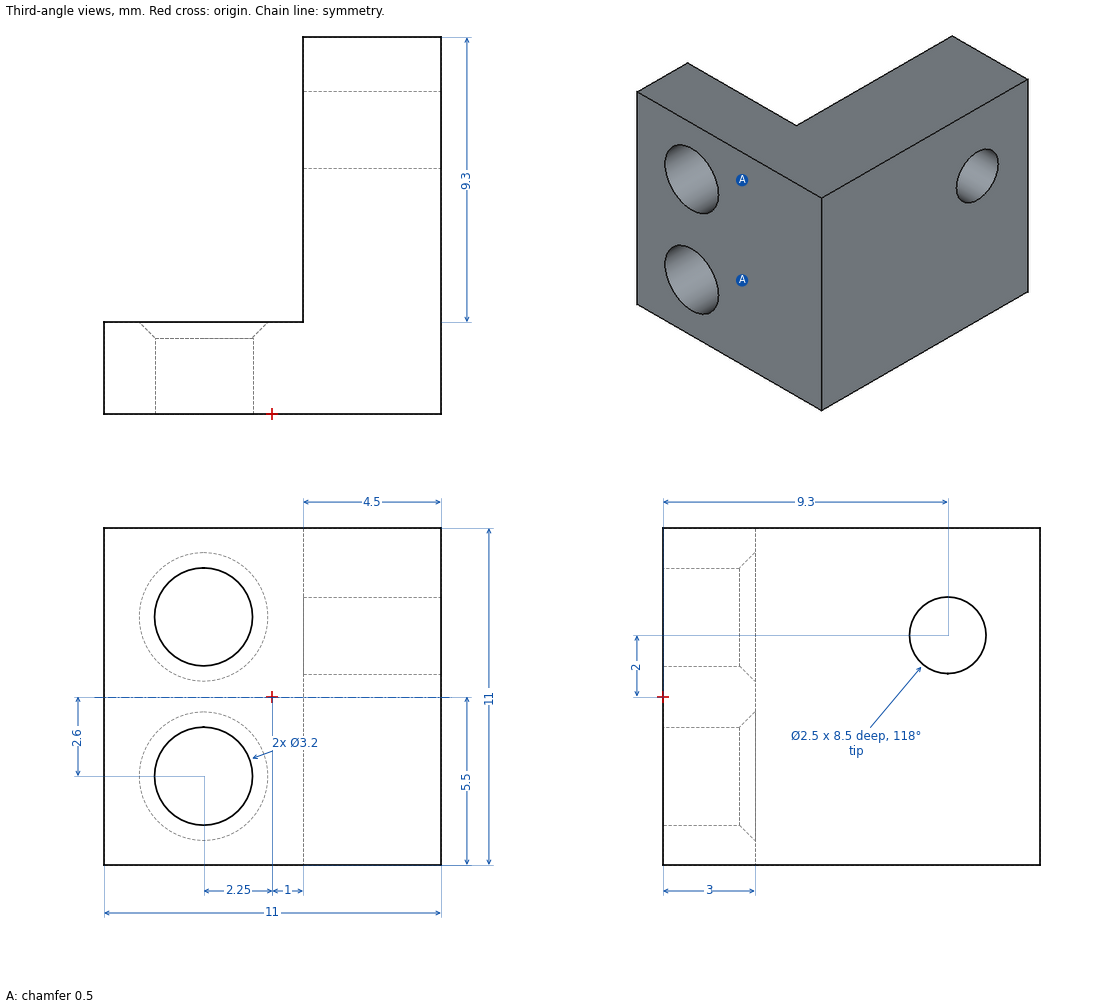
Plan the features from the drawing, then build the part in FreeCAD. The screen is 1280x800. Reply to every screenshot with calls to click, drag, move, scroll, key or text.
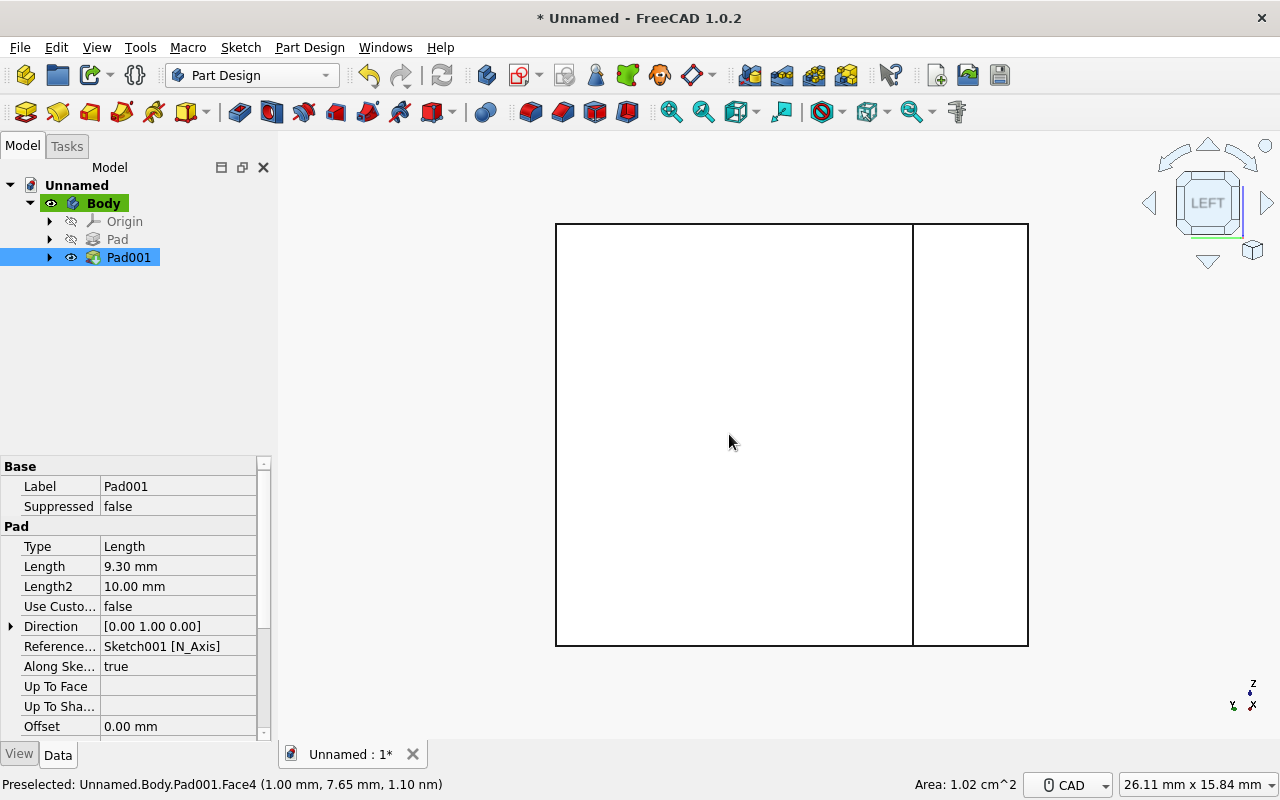
click(520, 76)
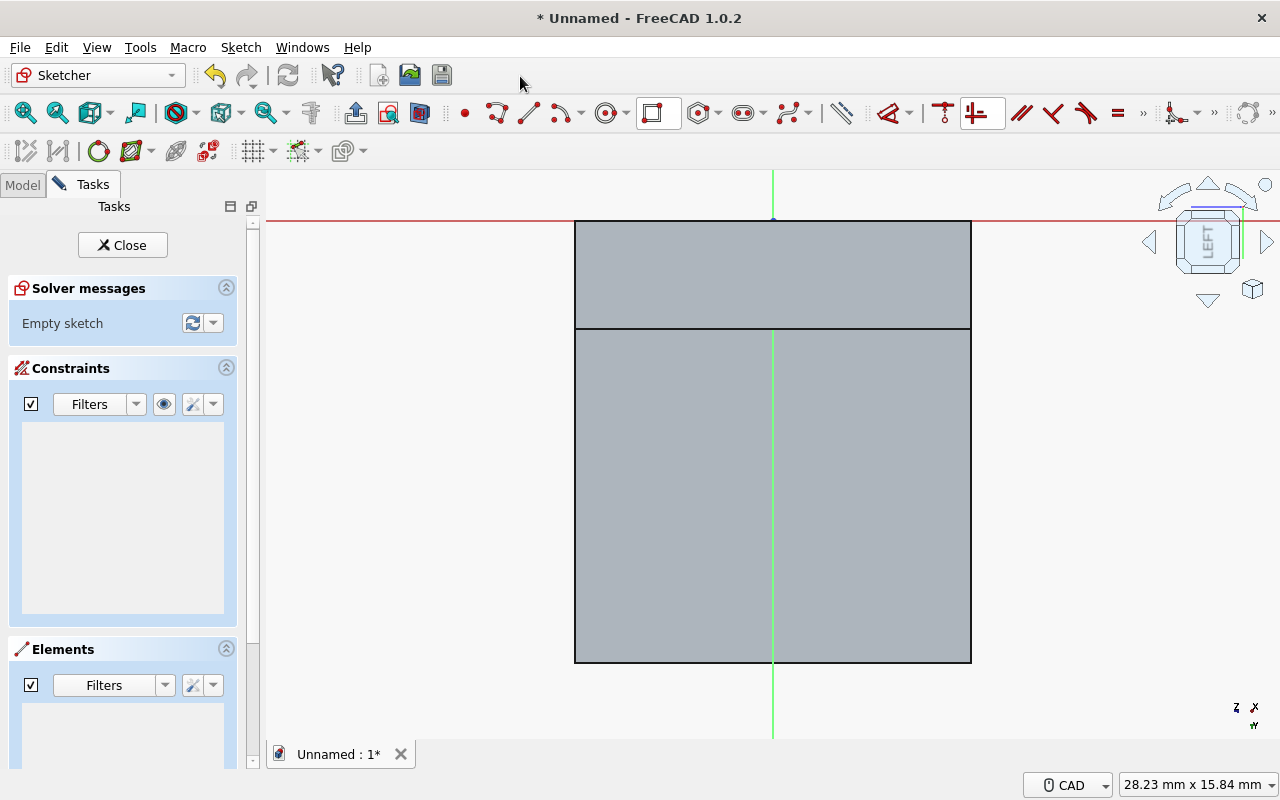
click(420, 114)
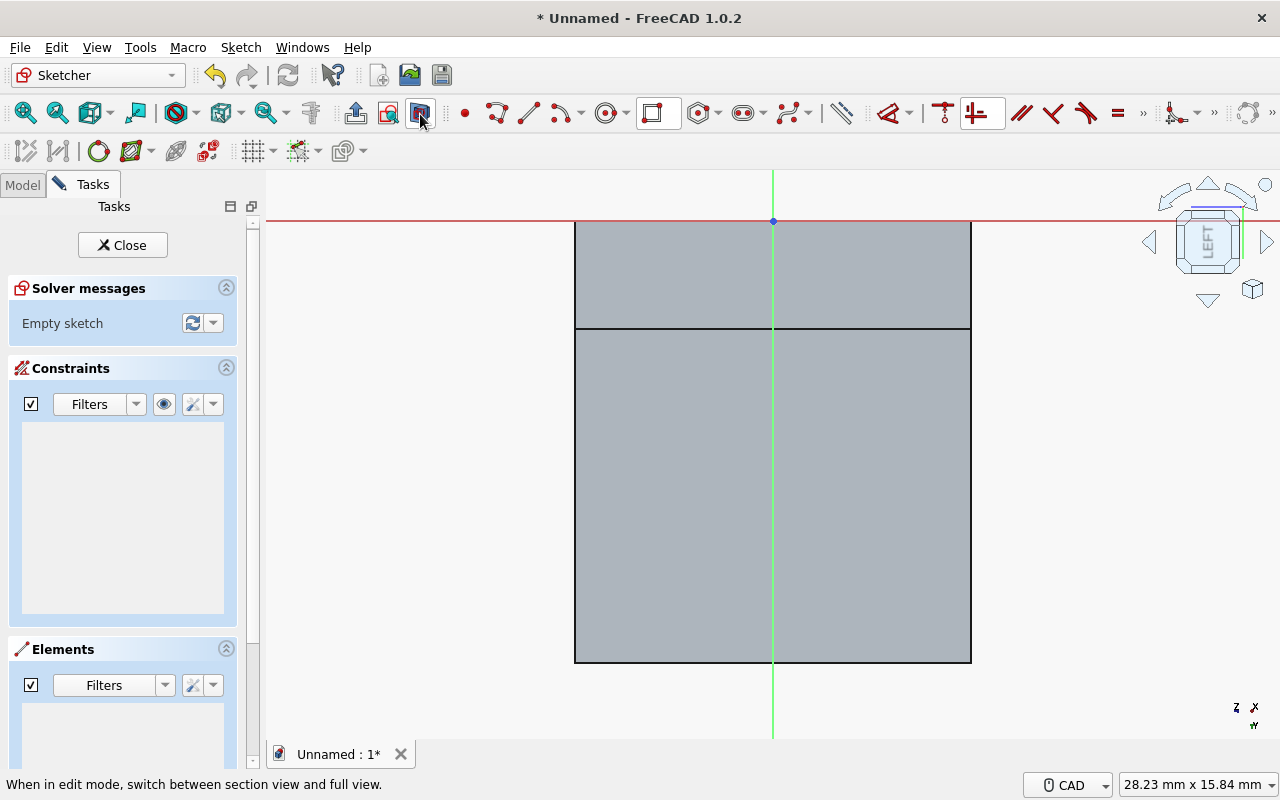
scroll(700, 588, up, 7)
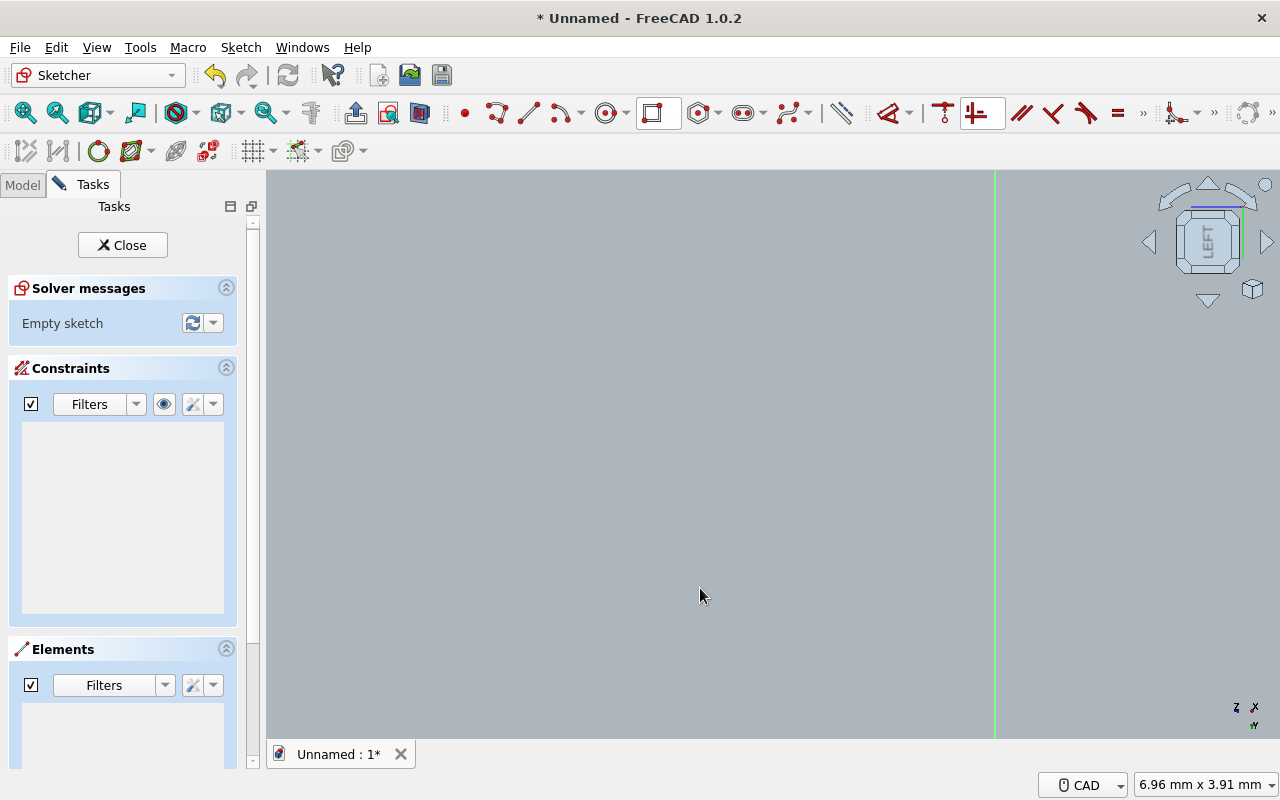
click(606, 114)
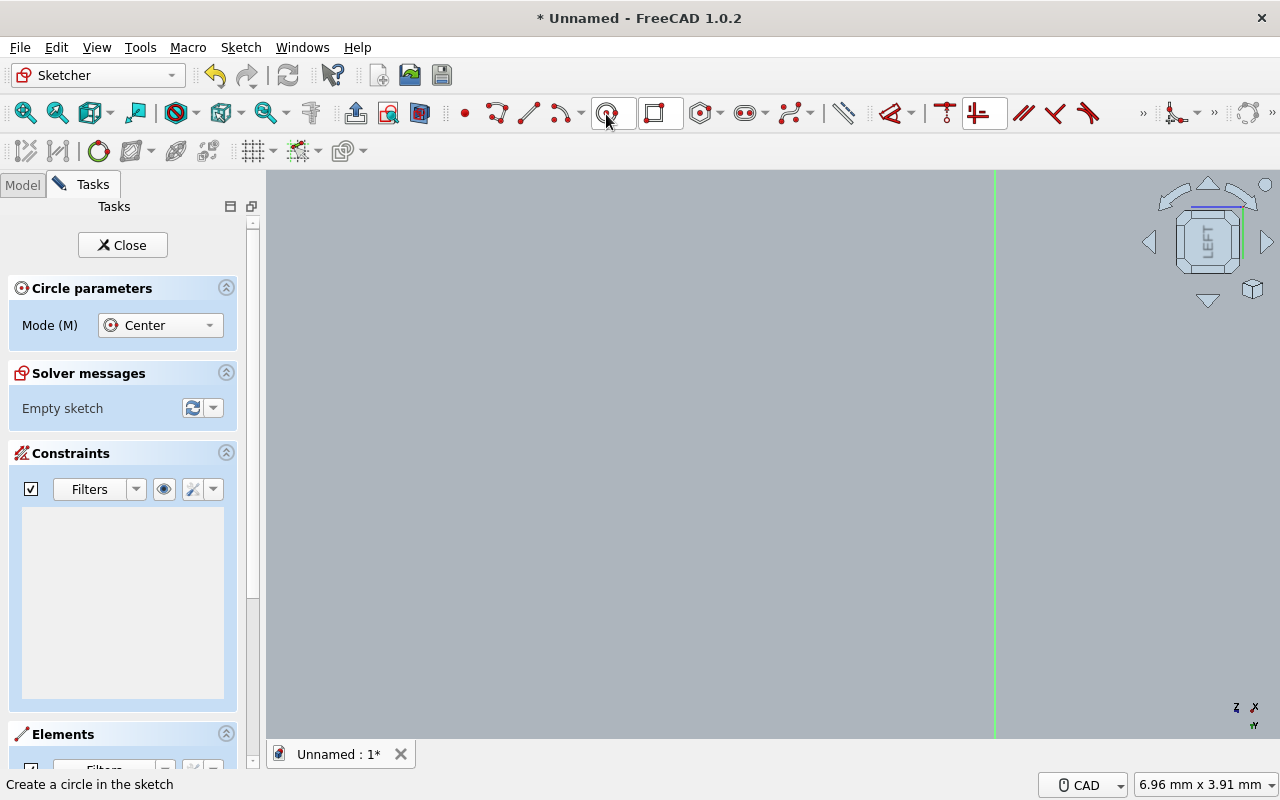
click(703, 452)
click(832, 323)
key(Escape)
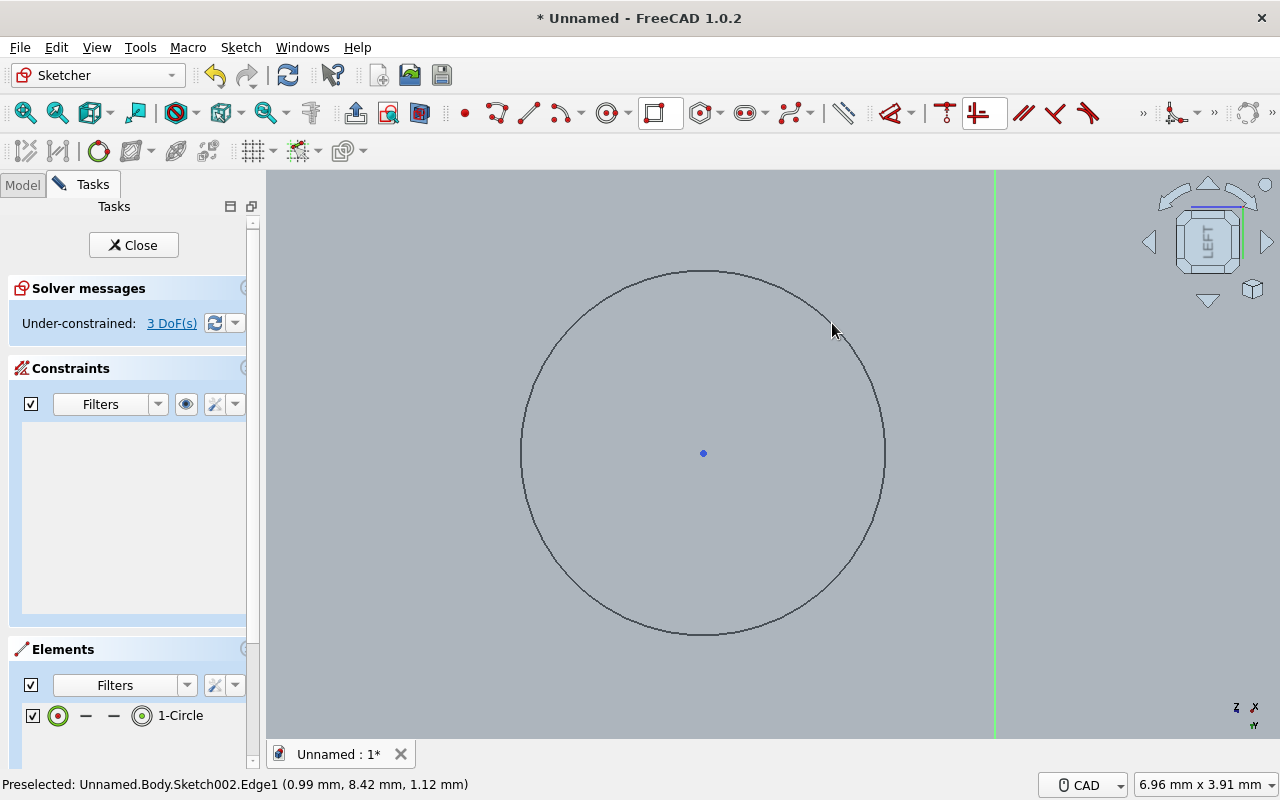
click(890, 114)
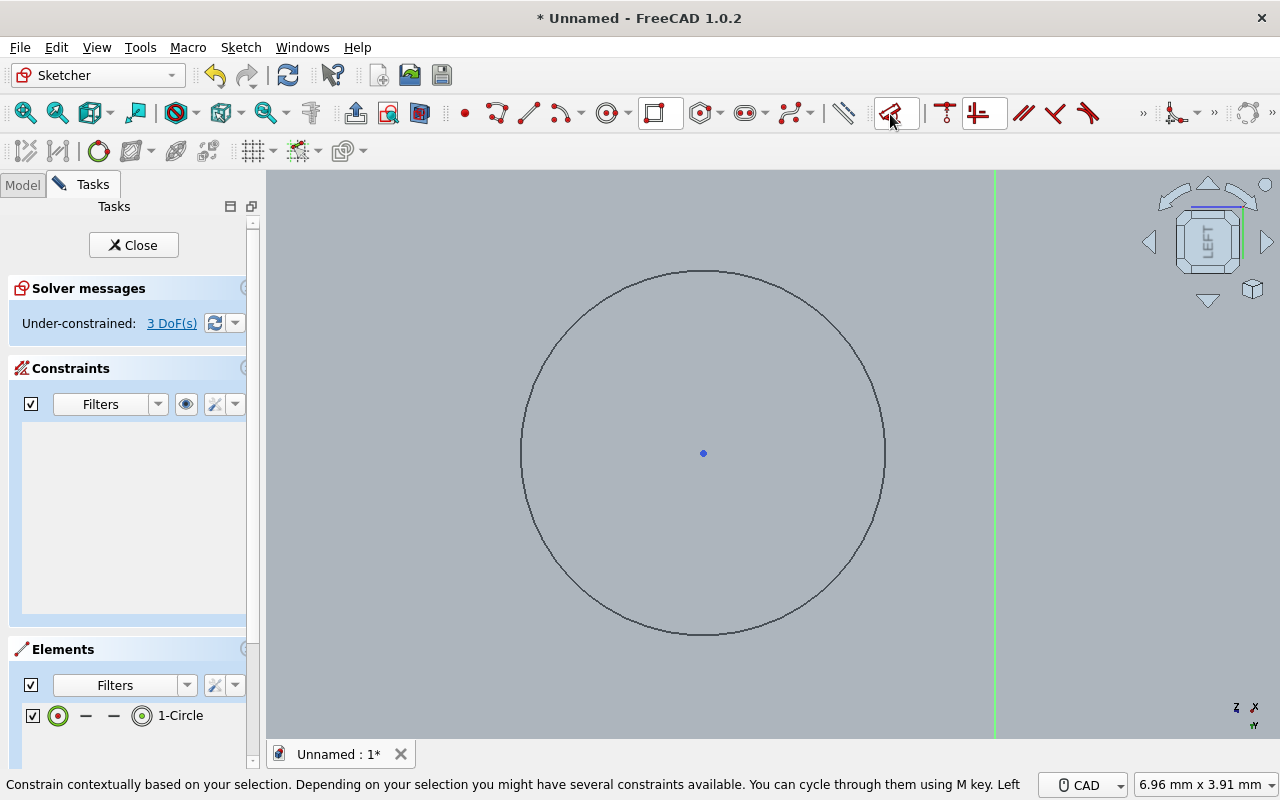
click(832, 324)
click(855, 301)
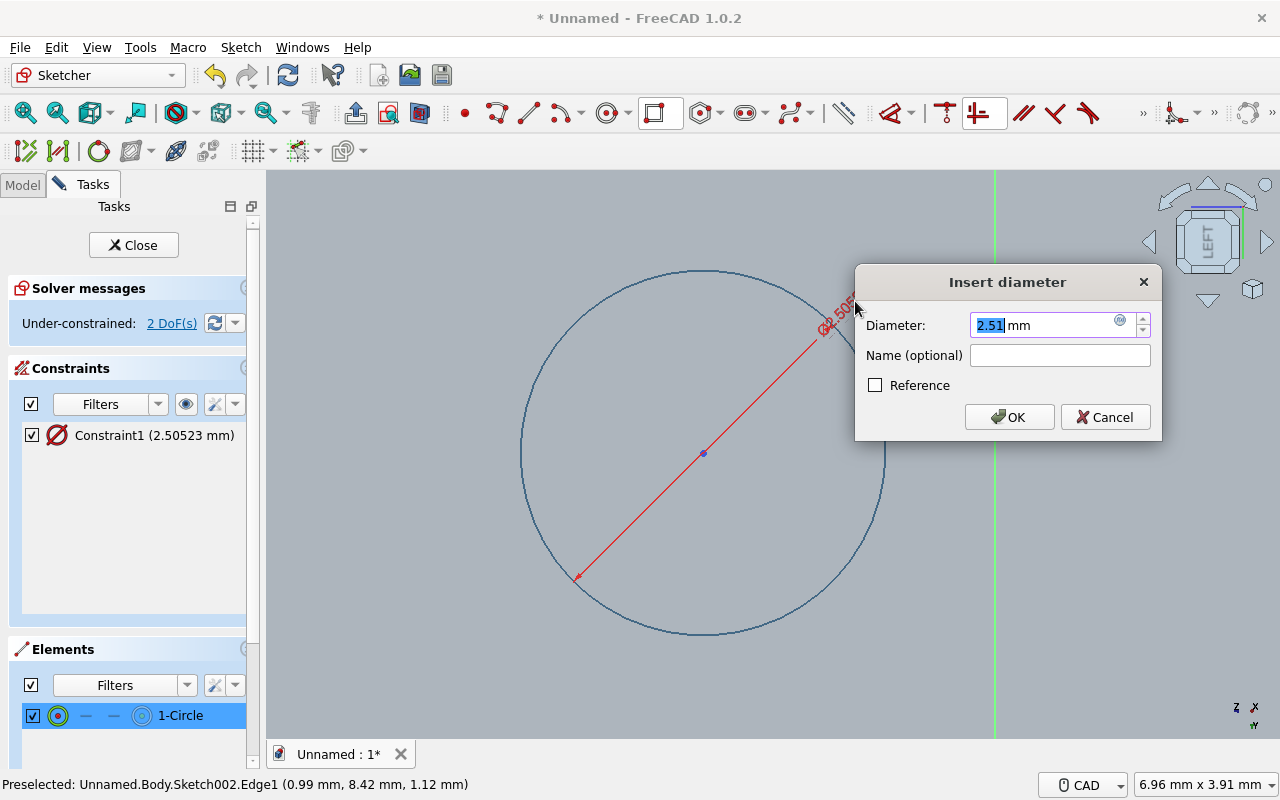
text(2.5)
key(Return)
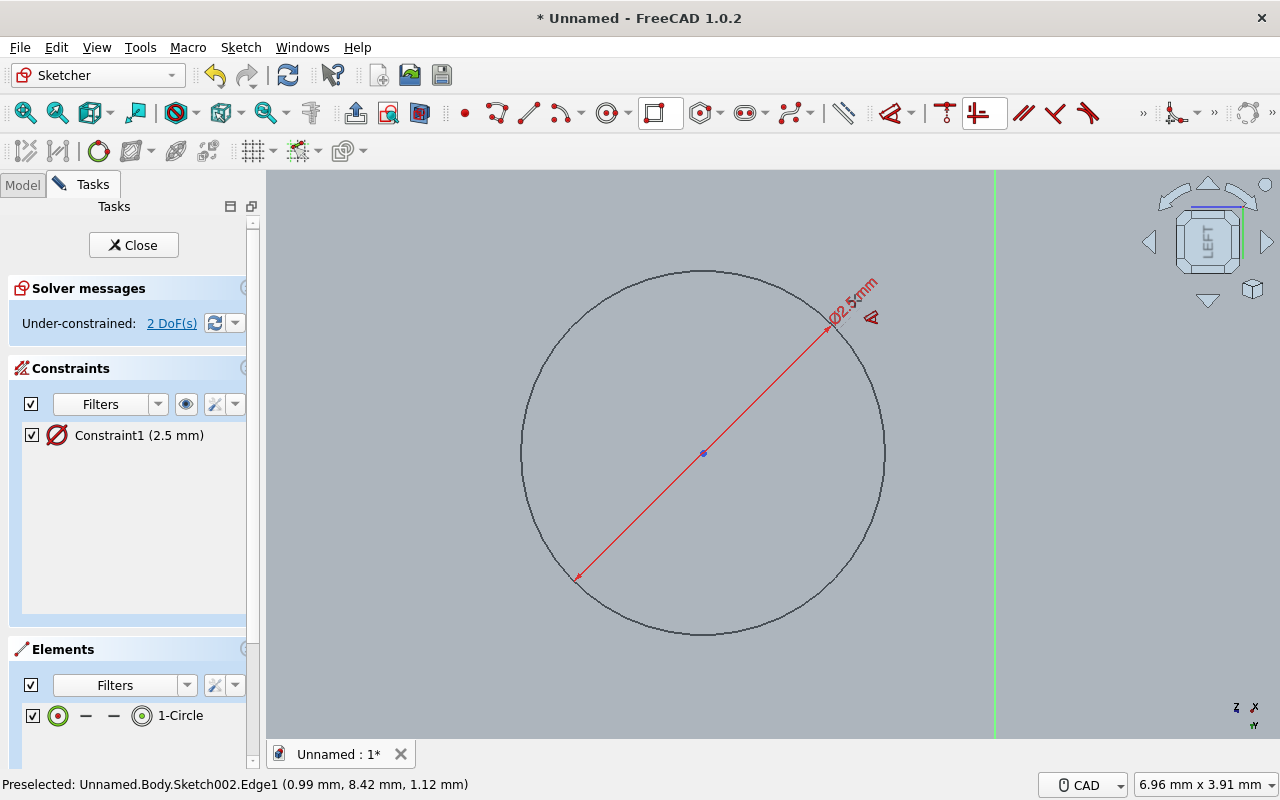
click(703, 453)
click(849, 487)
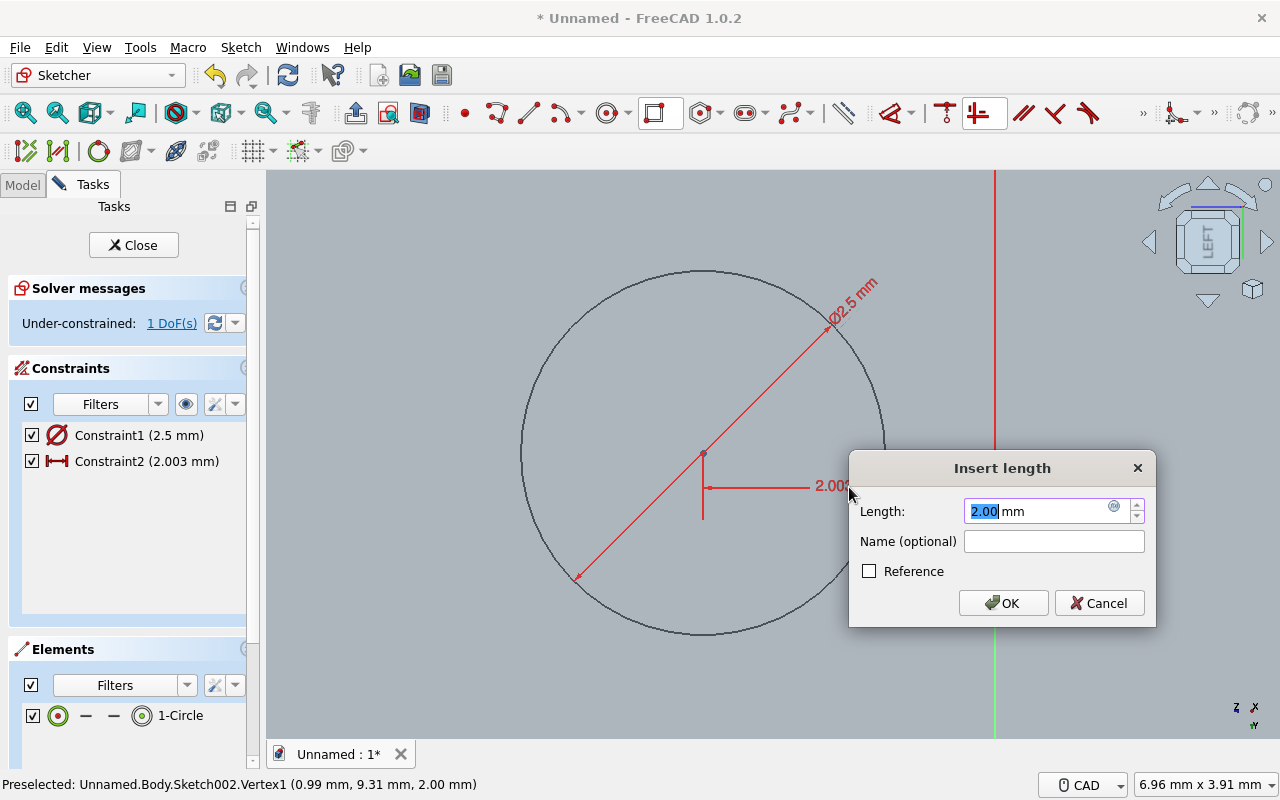
text(2)
key(Return)